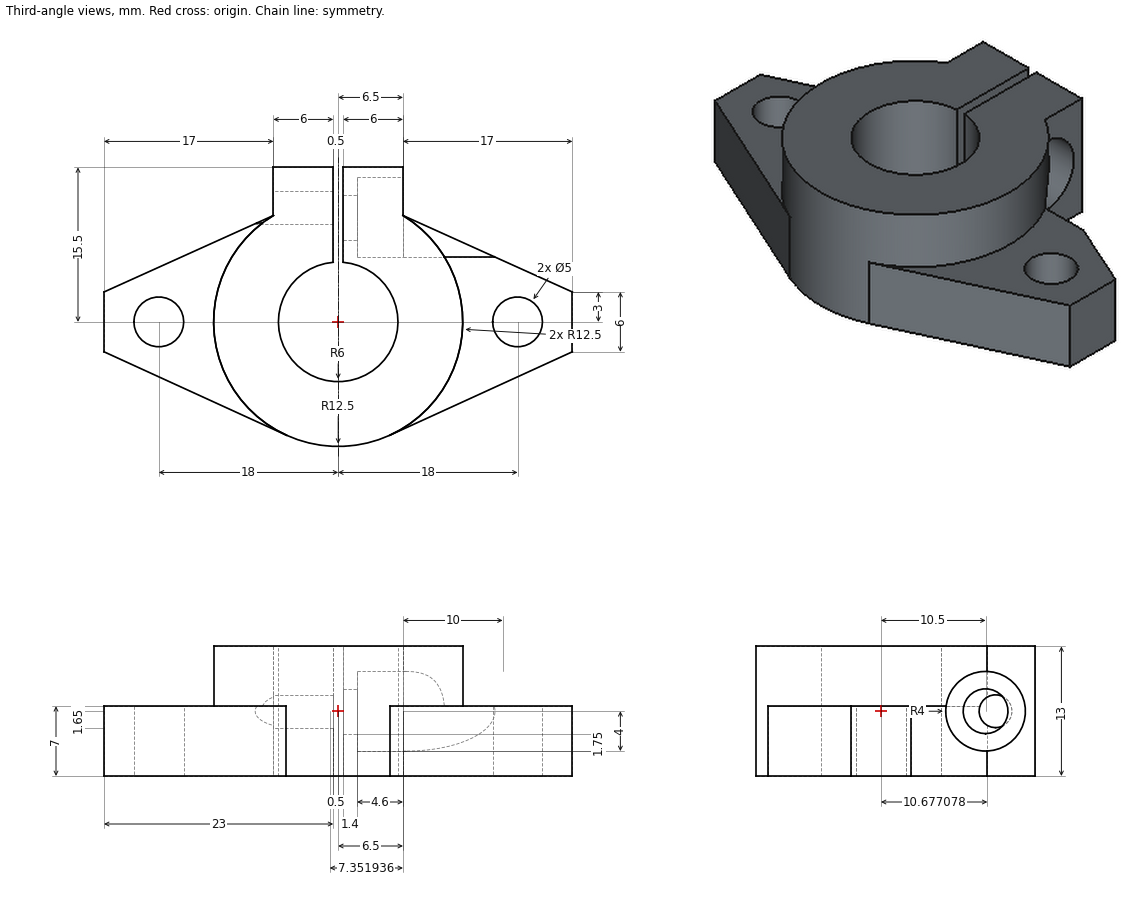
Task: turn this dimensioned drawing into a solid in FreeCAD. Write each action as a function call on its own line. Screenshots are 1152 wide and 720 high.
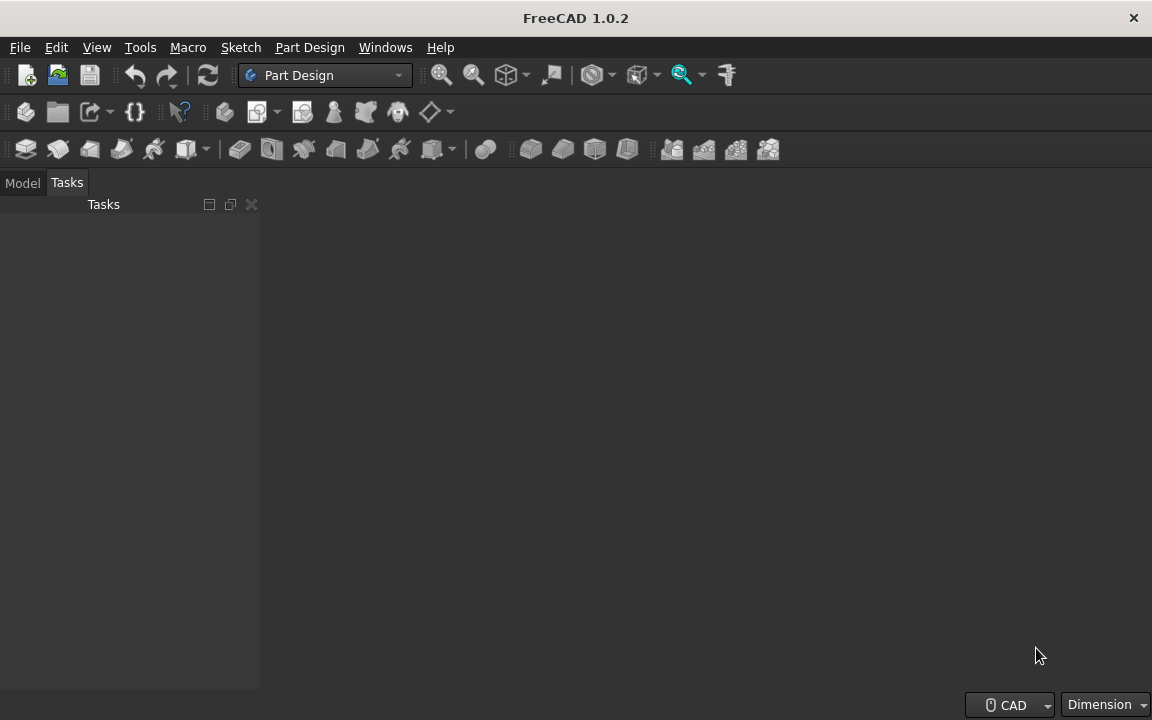
click(26, 76)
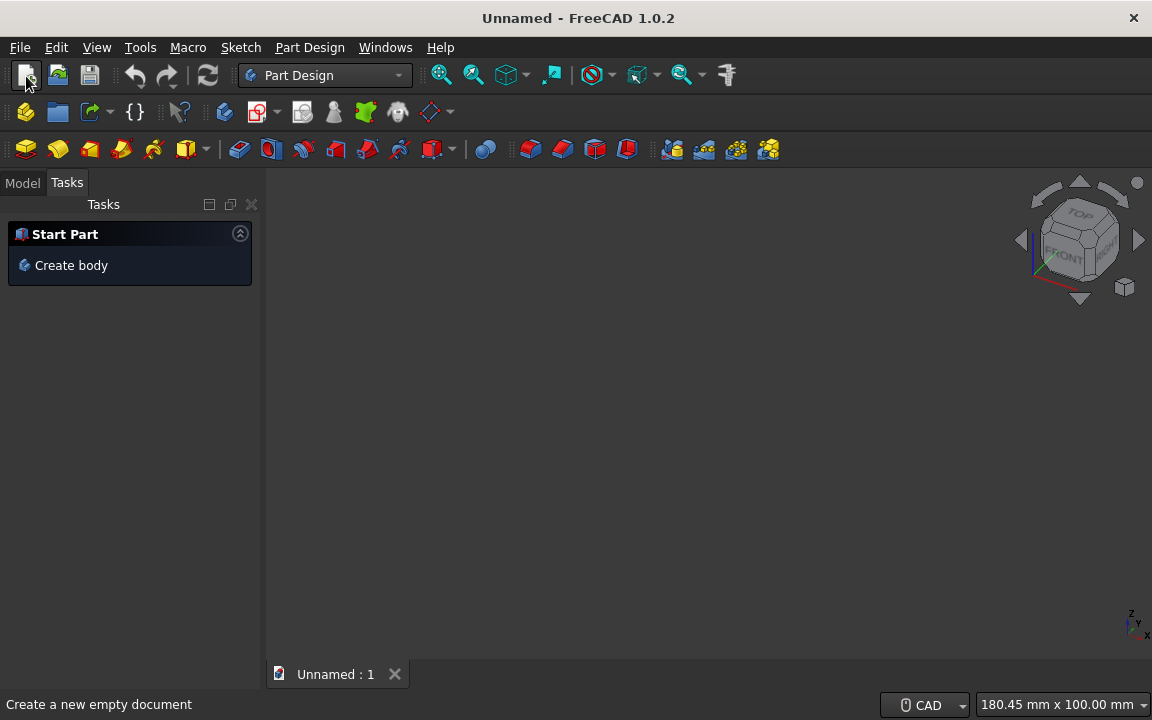
click(258, 112)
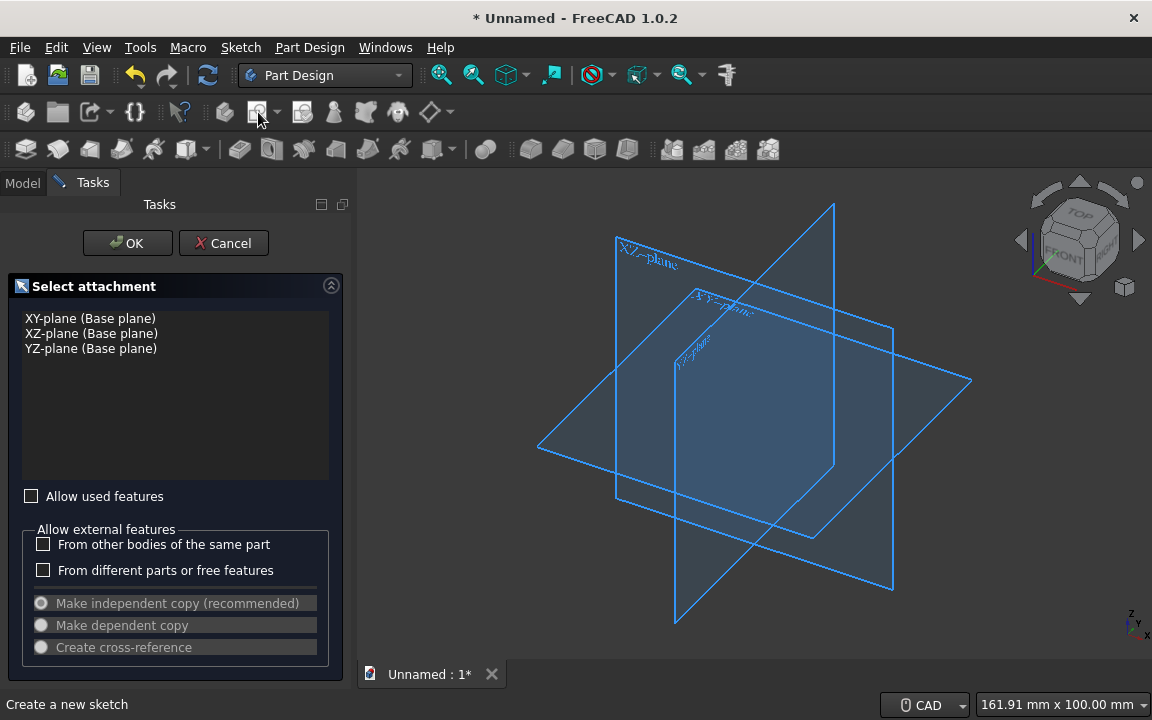
click(82, 318)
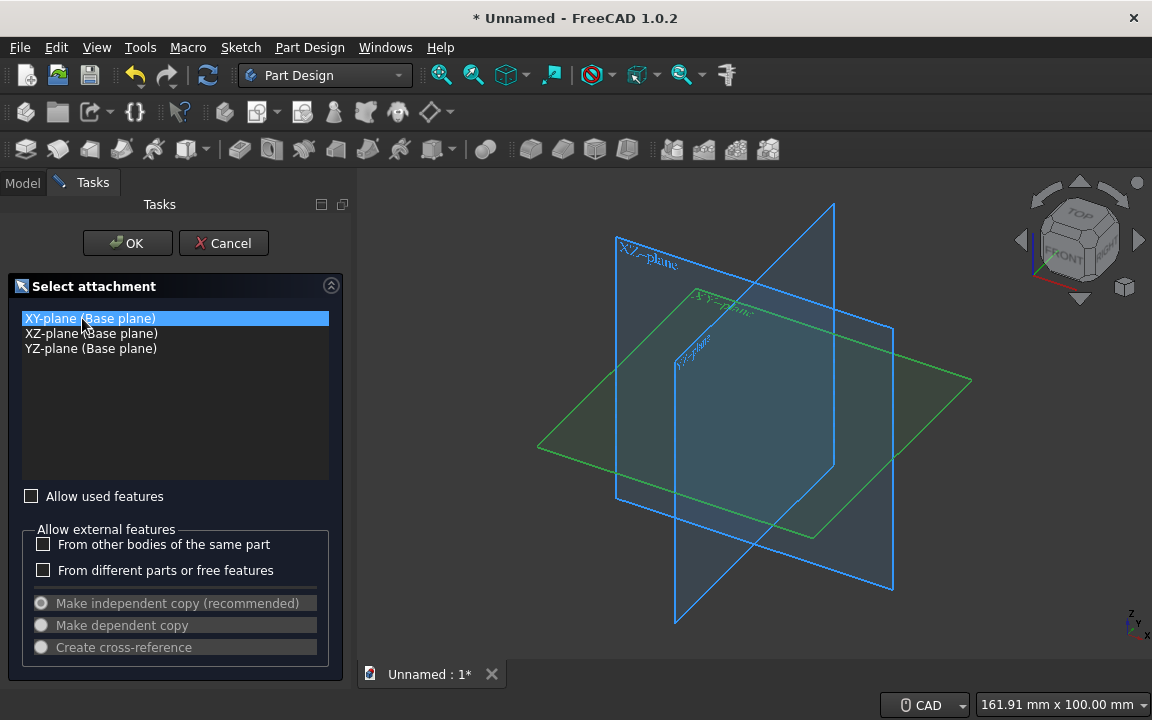
click(128, 243)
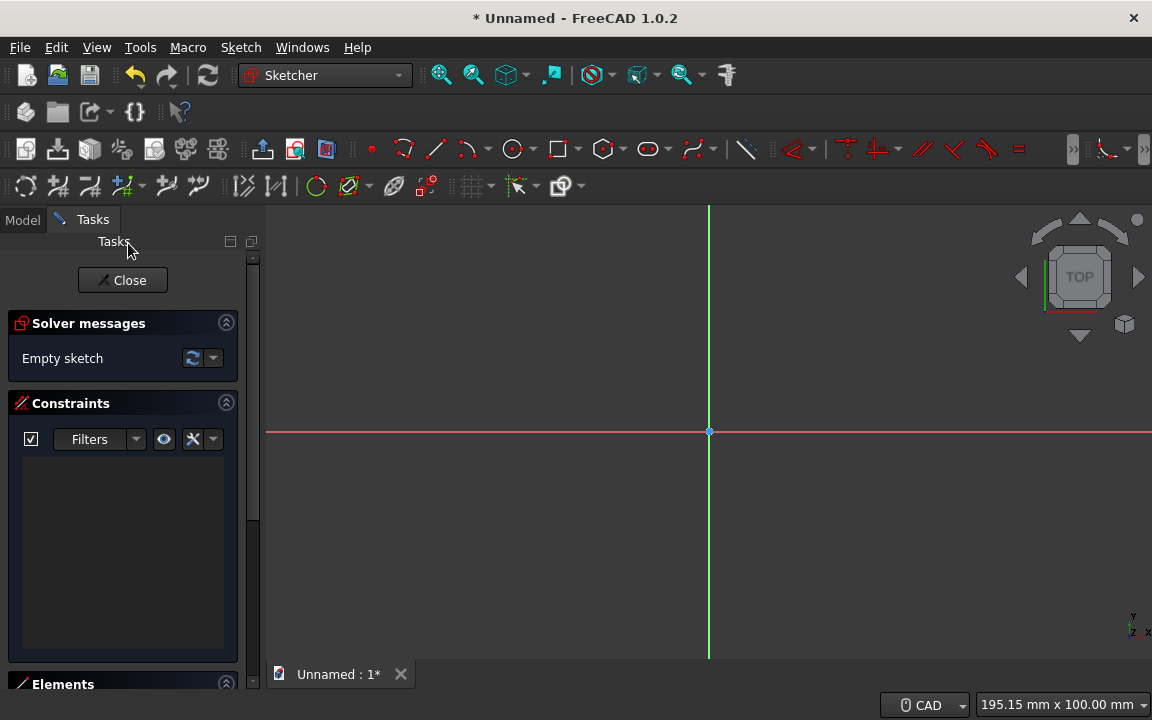
scroll(765, 420, up, 4)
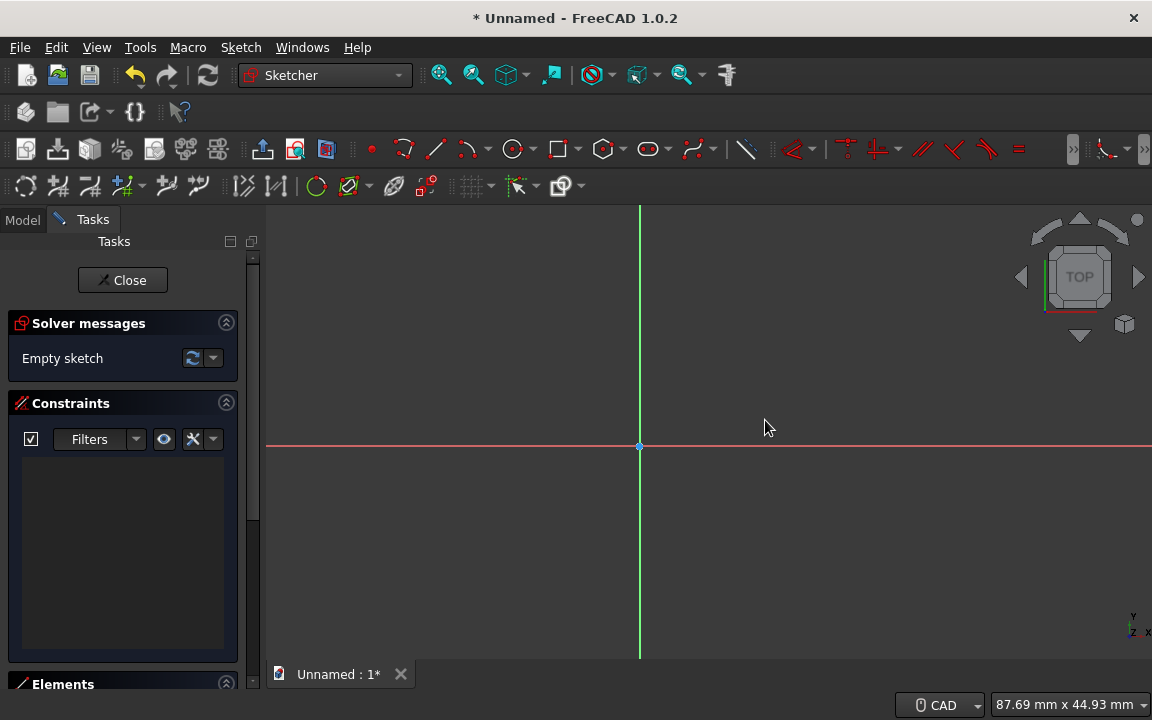
click(404, 150)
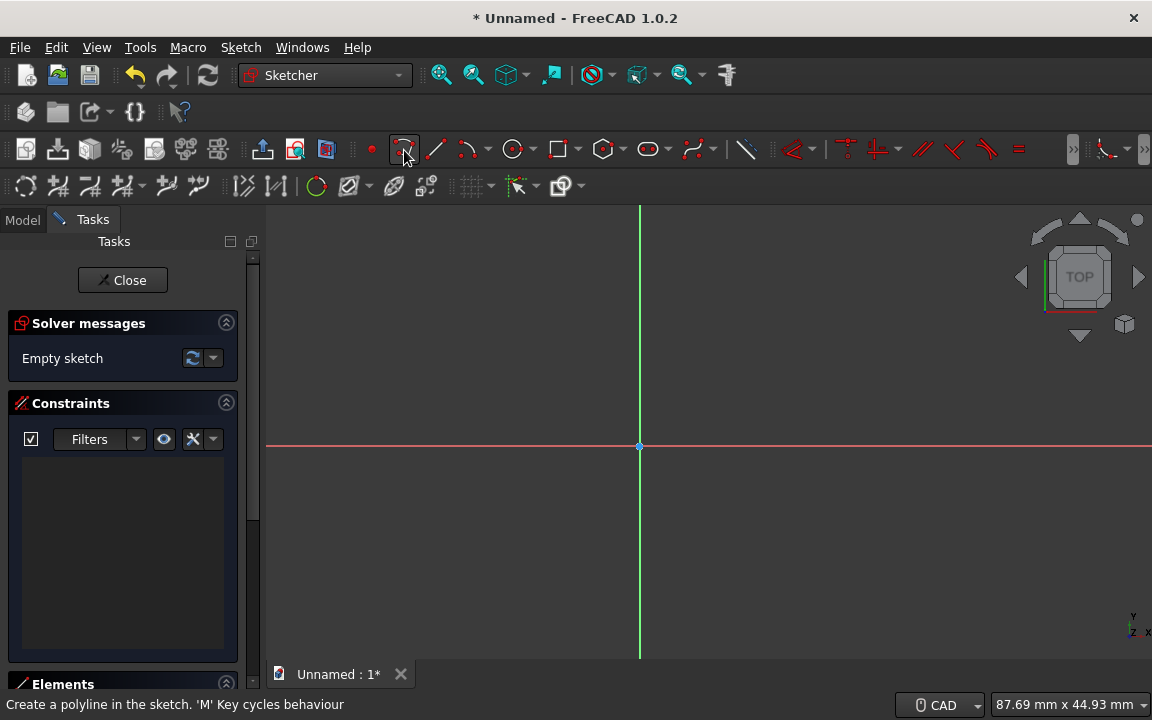
scroll(635, 386, up, 6)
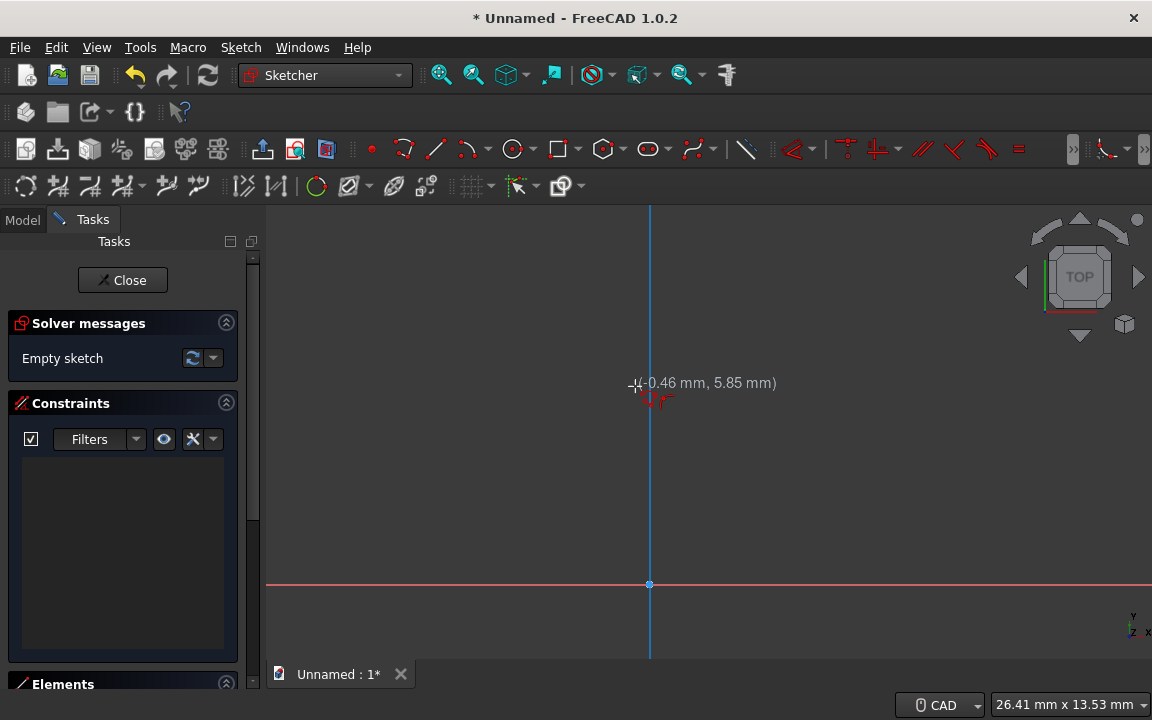
click(633, 384)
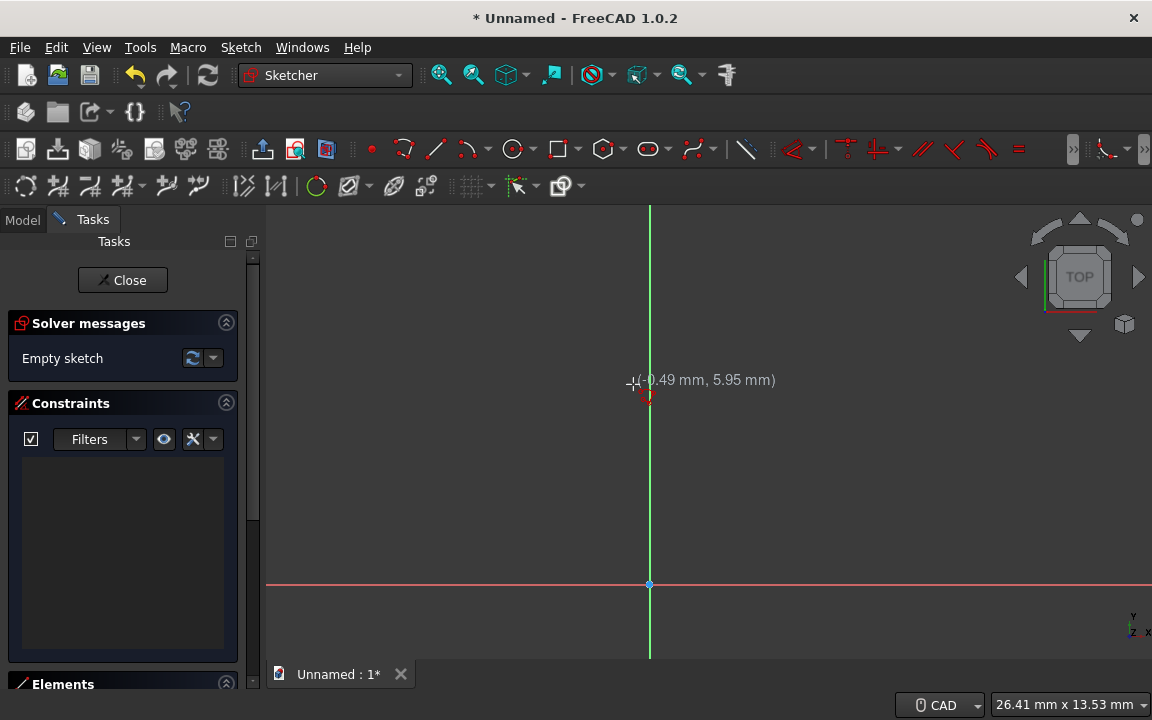
scroll(637, 388, down, 6)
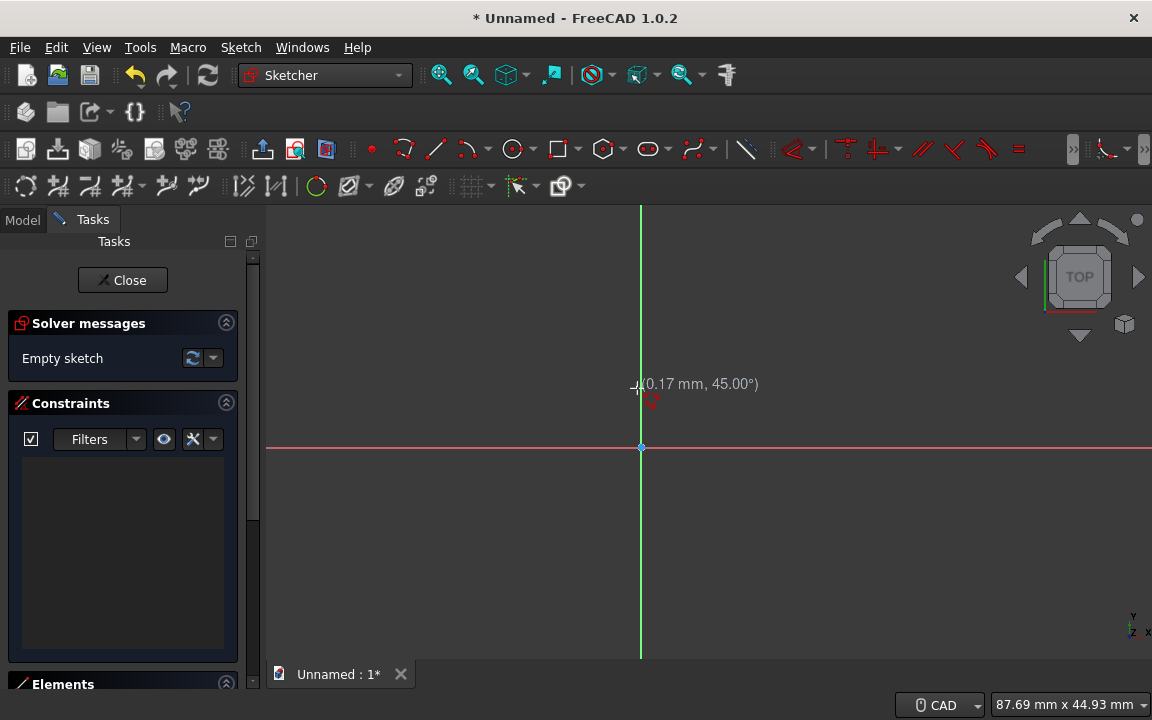
scroll(636, 291, up, 6)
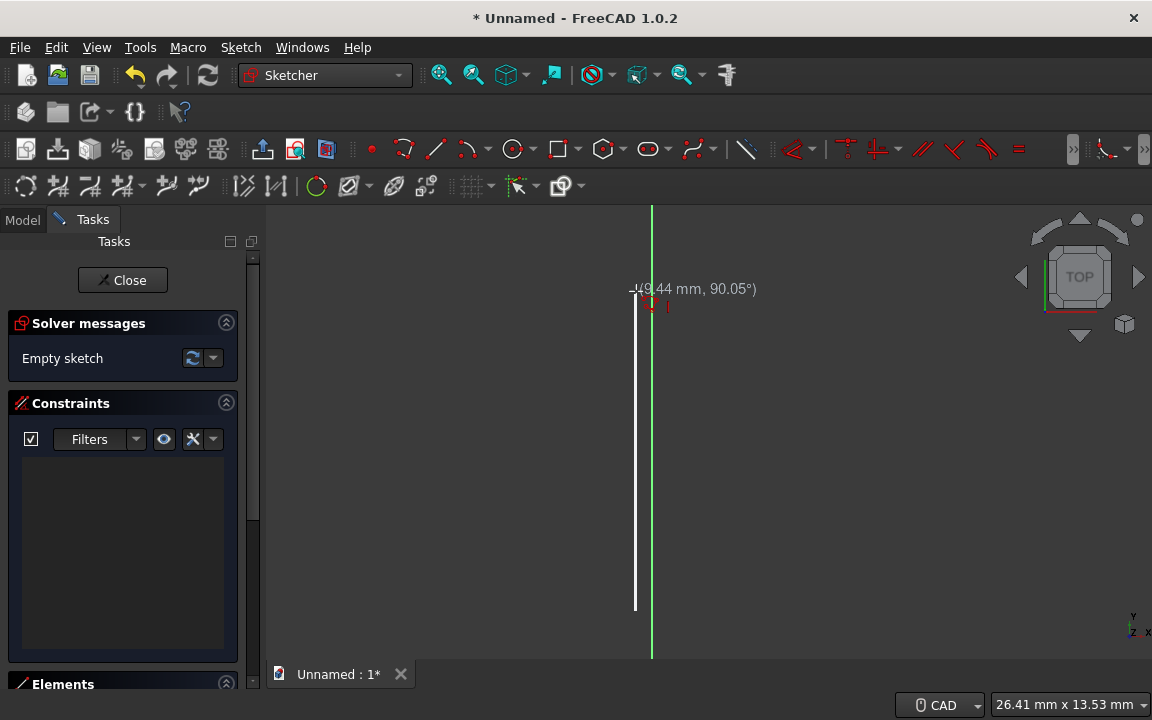
click(635, 290)
click(434, 290)
click(434, 452)
right_click(434, 452)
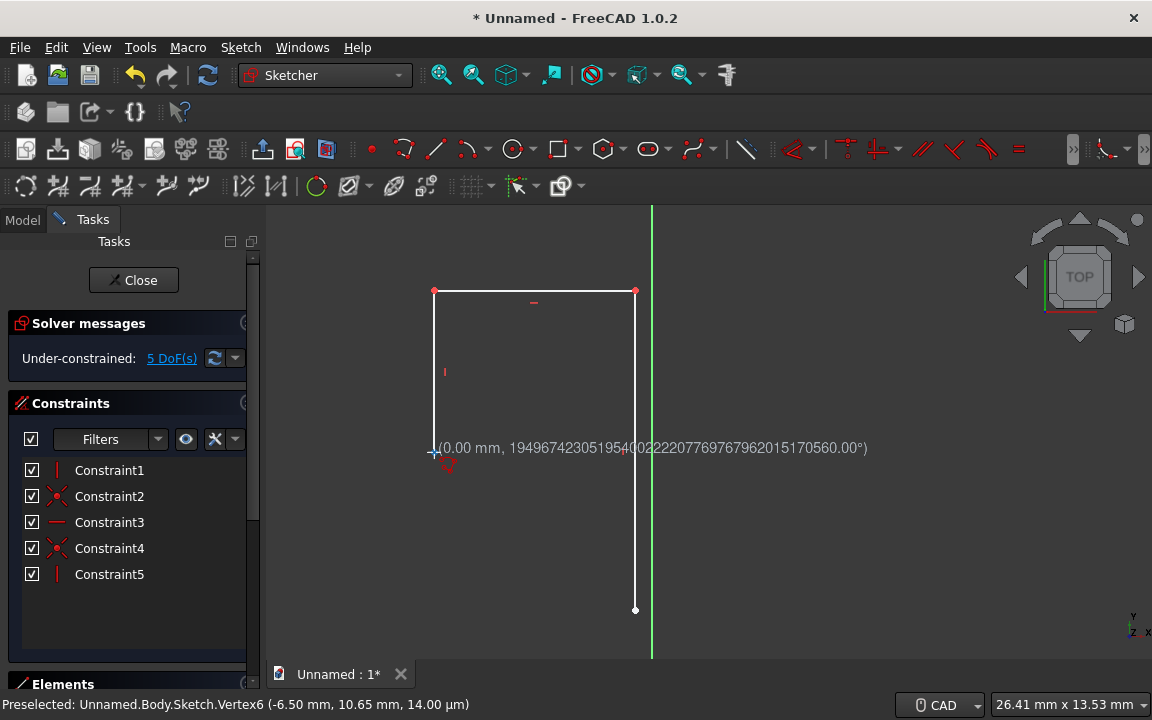
click(870, 452)
click(870, 290)
click(669, 290)
click(669, 610)
right_click(669, 610)